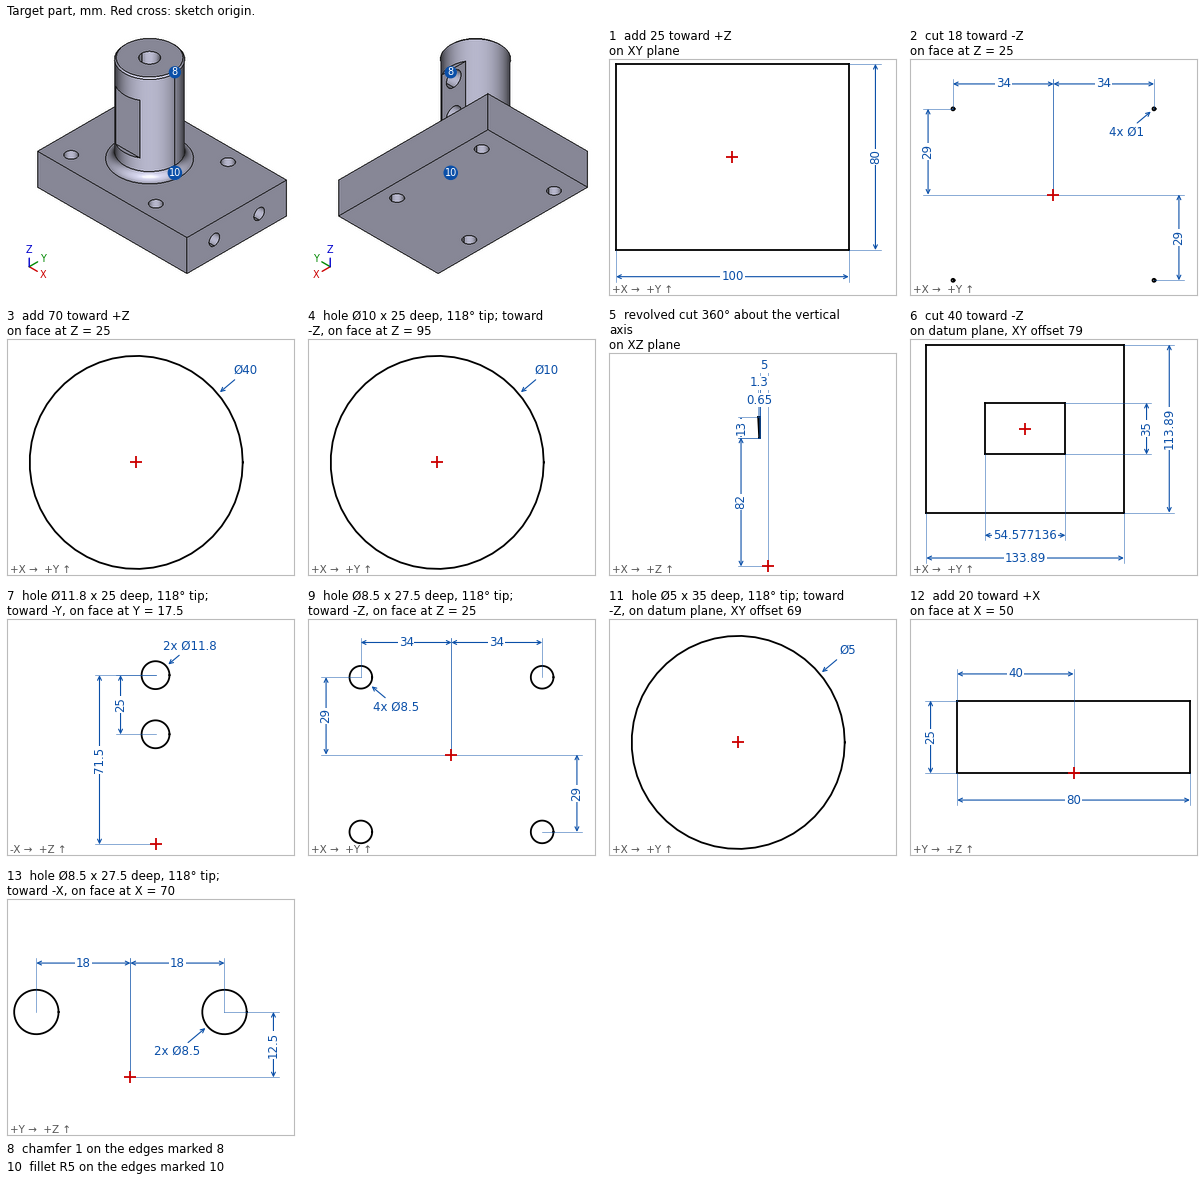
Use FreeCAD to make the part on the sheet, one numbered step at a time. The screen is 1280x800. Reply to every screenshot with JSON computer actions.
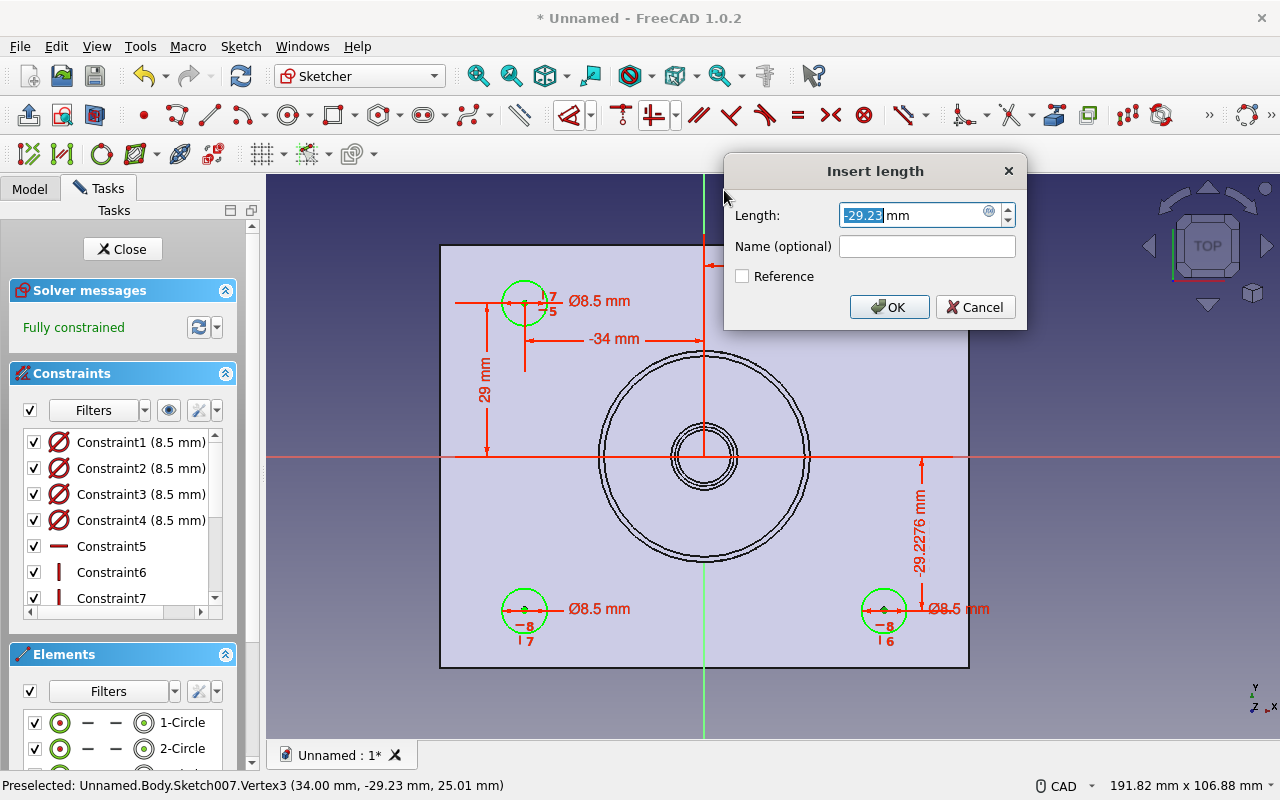
{"action": "type", "text": "-29"}
{"action": "key", "text": "Return"}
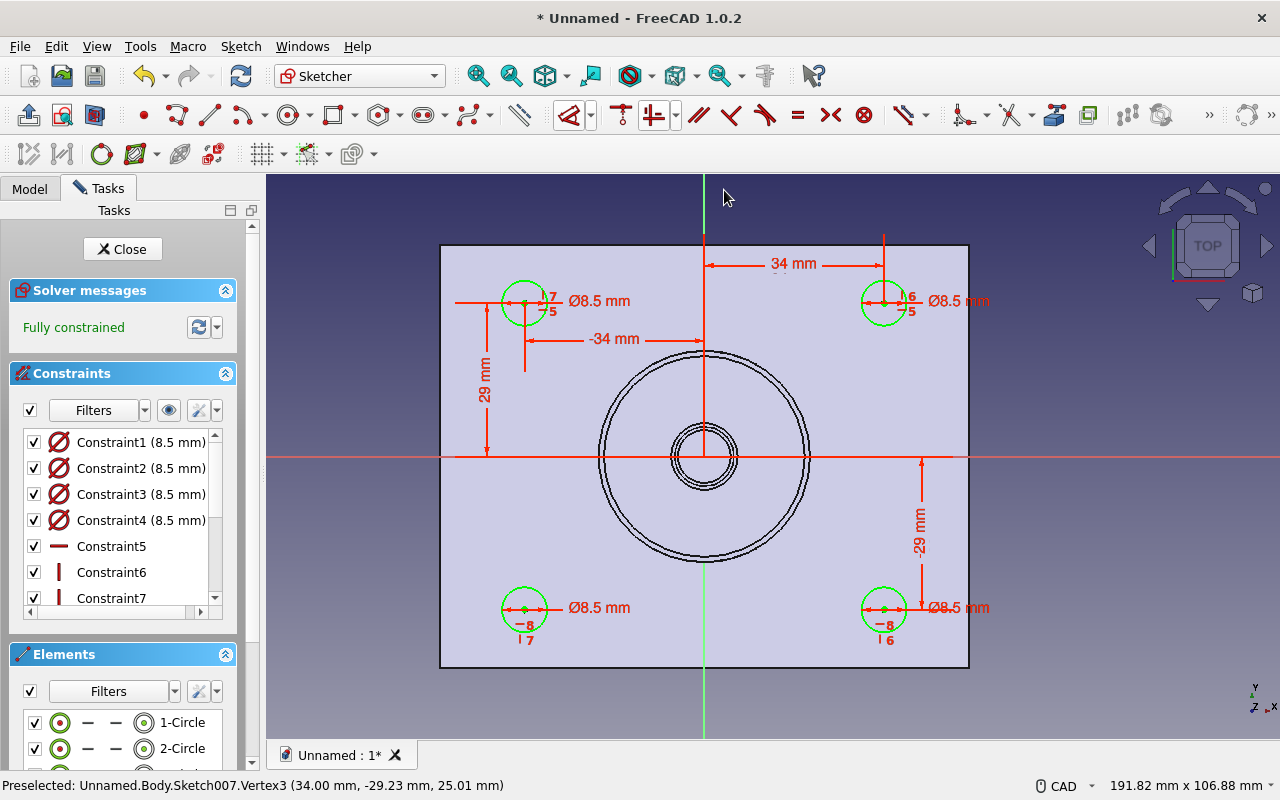
{"action": "left_click", "coordinate": [123, 249]}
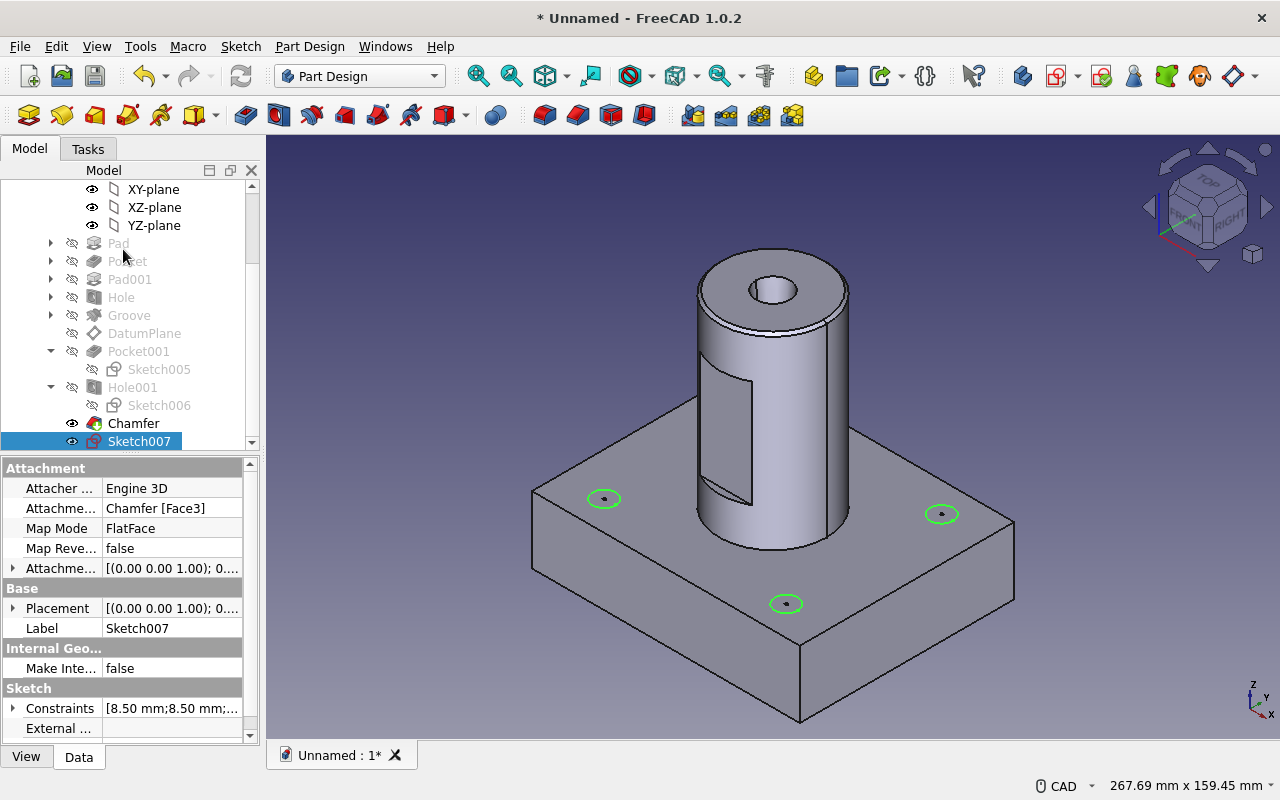
{"action": "left_click", "coordinate": [279, 116]}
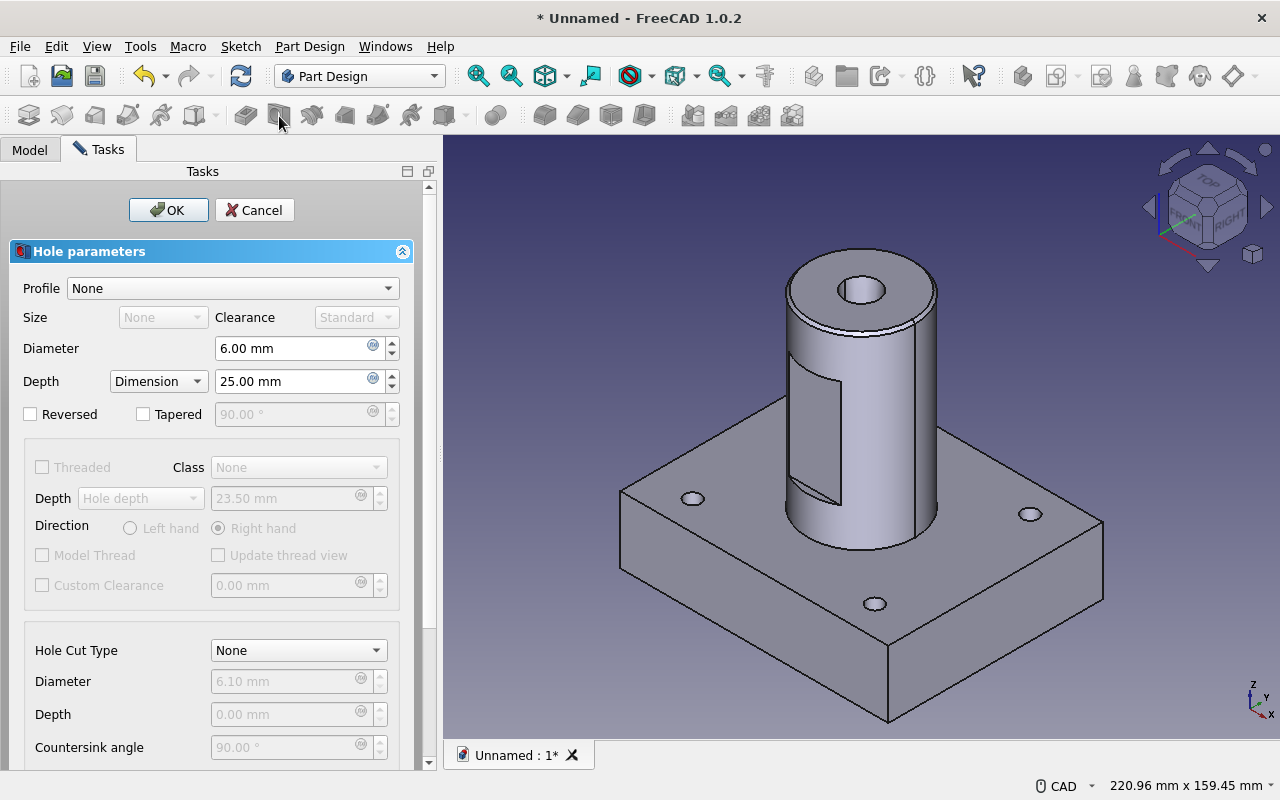
{"action": "triple_click", "coordinate": [300, 348]}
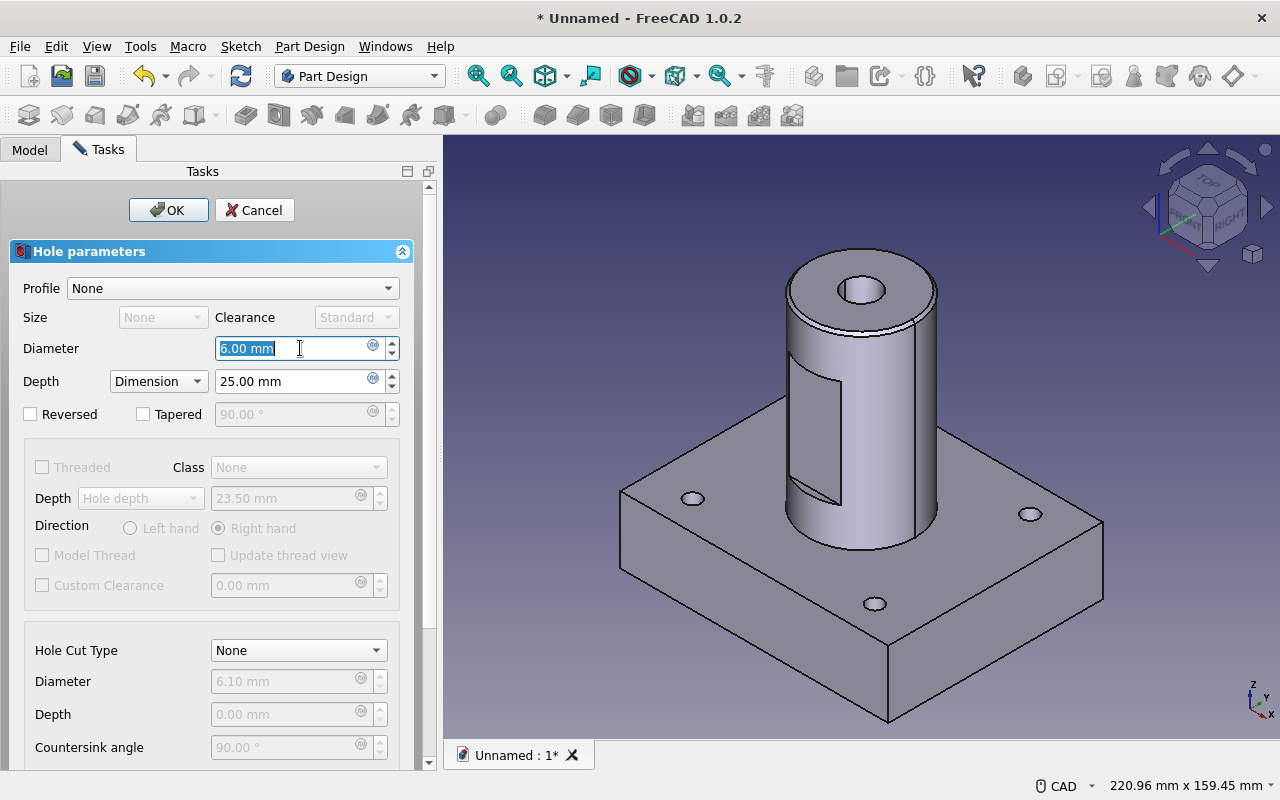
{"action": "type", "text": "8.5"}
{"action": "key", "text": "Tab"}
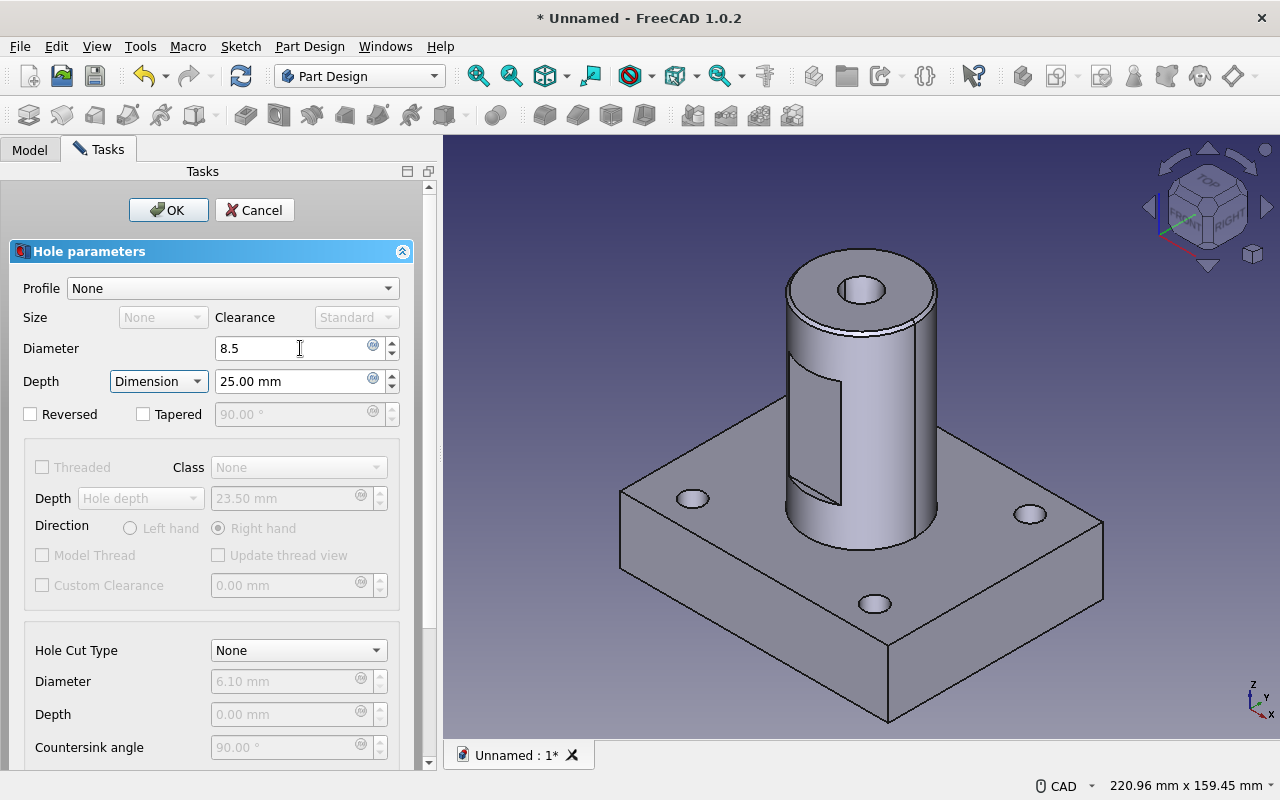
{"action": "triple_click", "coordinate": [300, 382]}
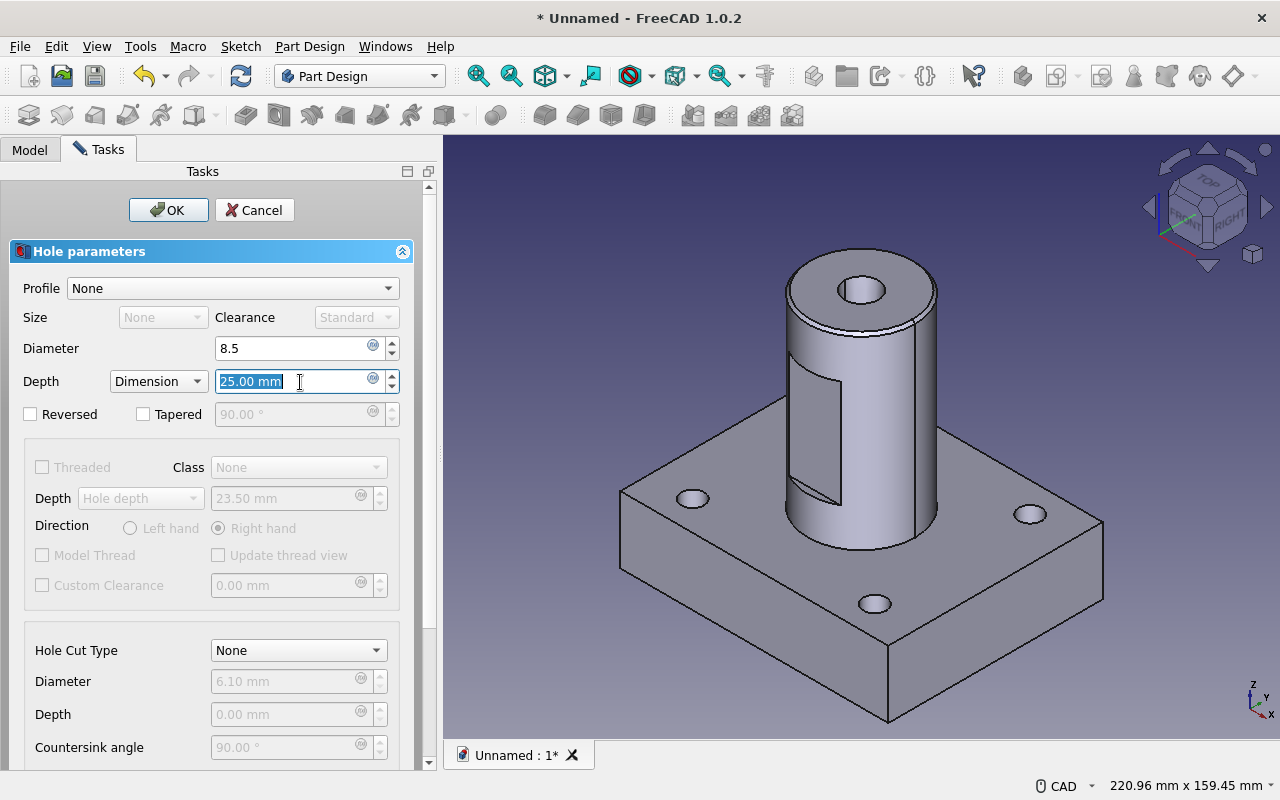
{"action": "type", "text": "27.5"}
{"action": "key", "text": "Tab"}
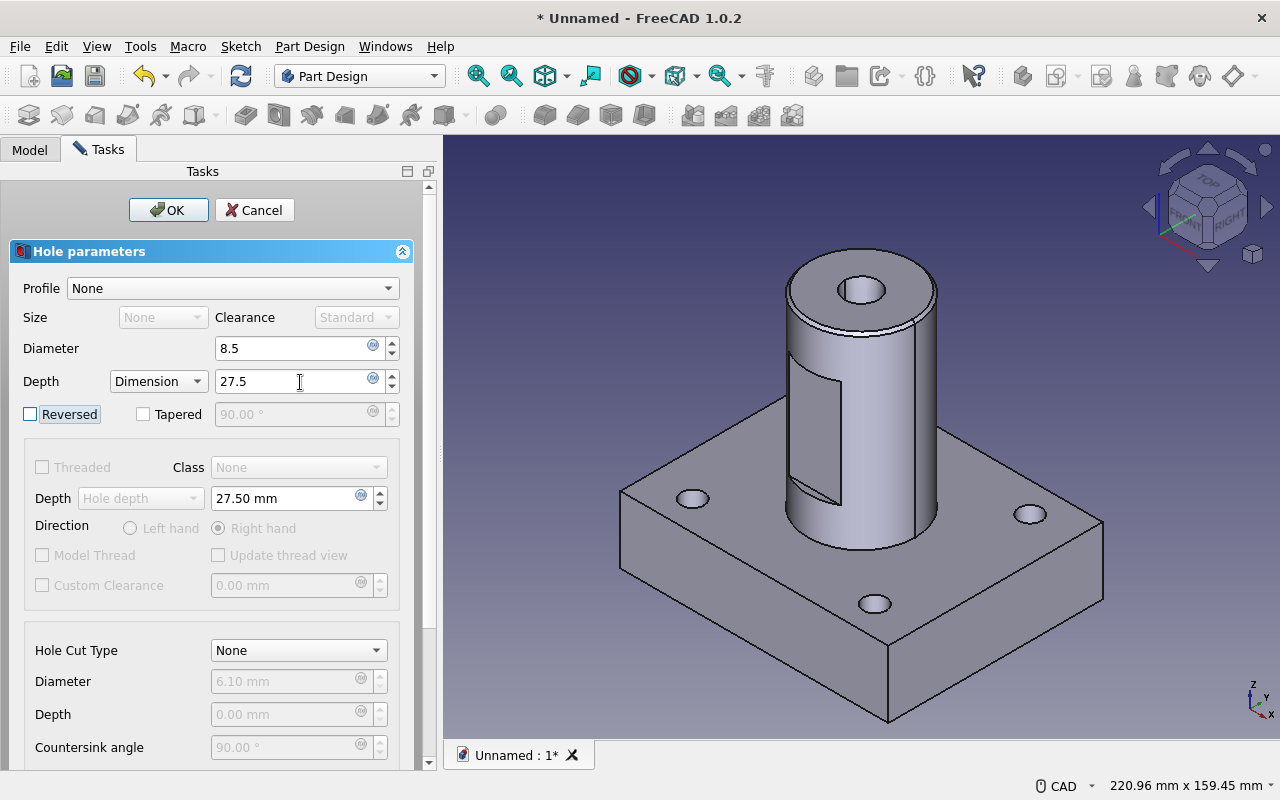
{"action": "left_click", "coordinate": [169, 210]}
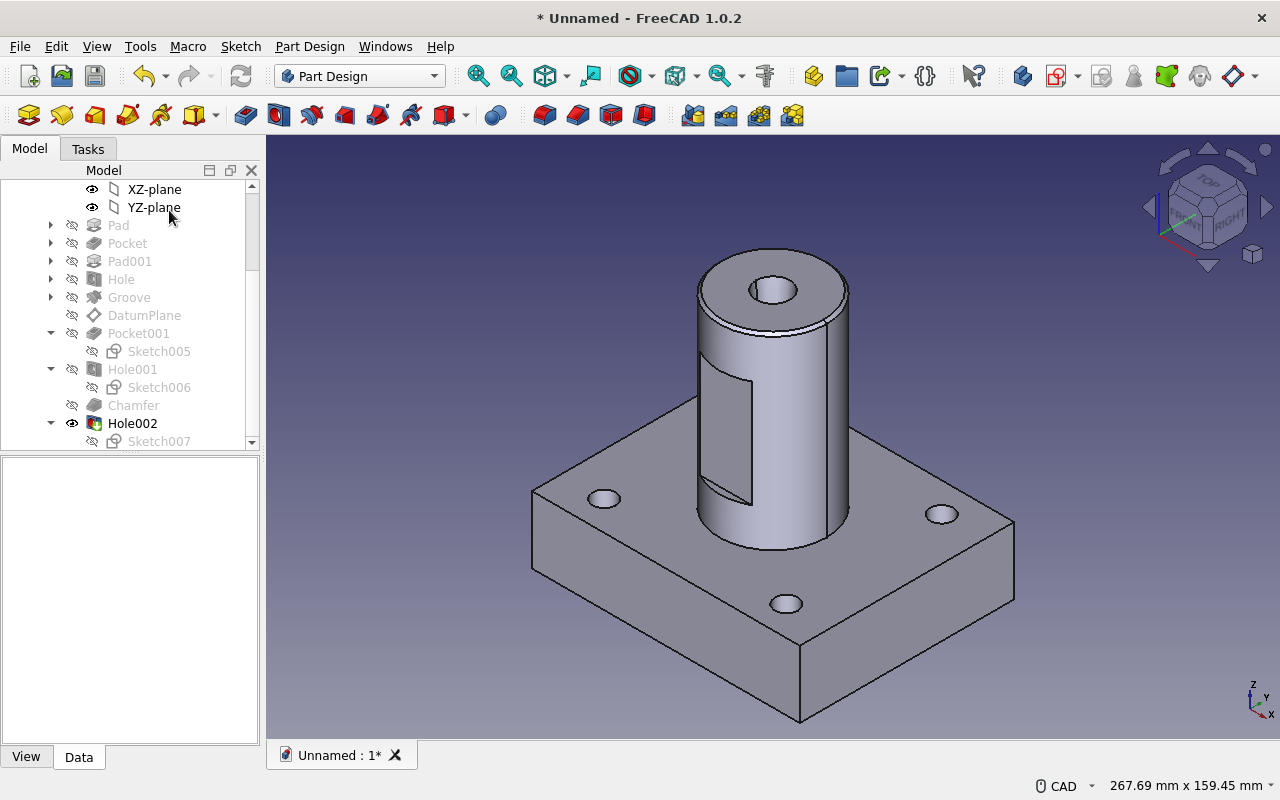
{"action": "key", "text": "2"}